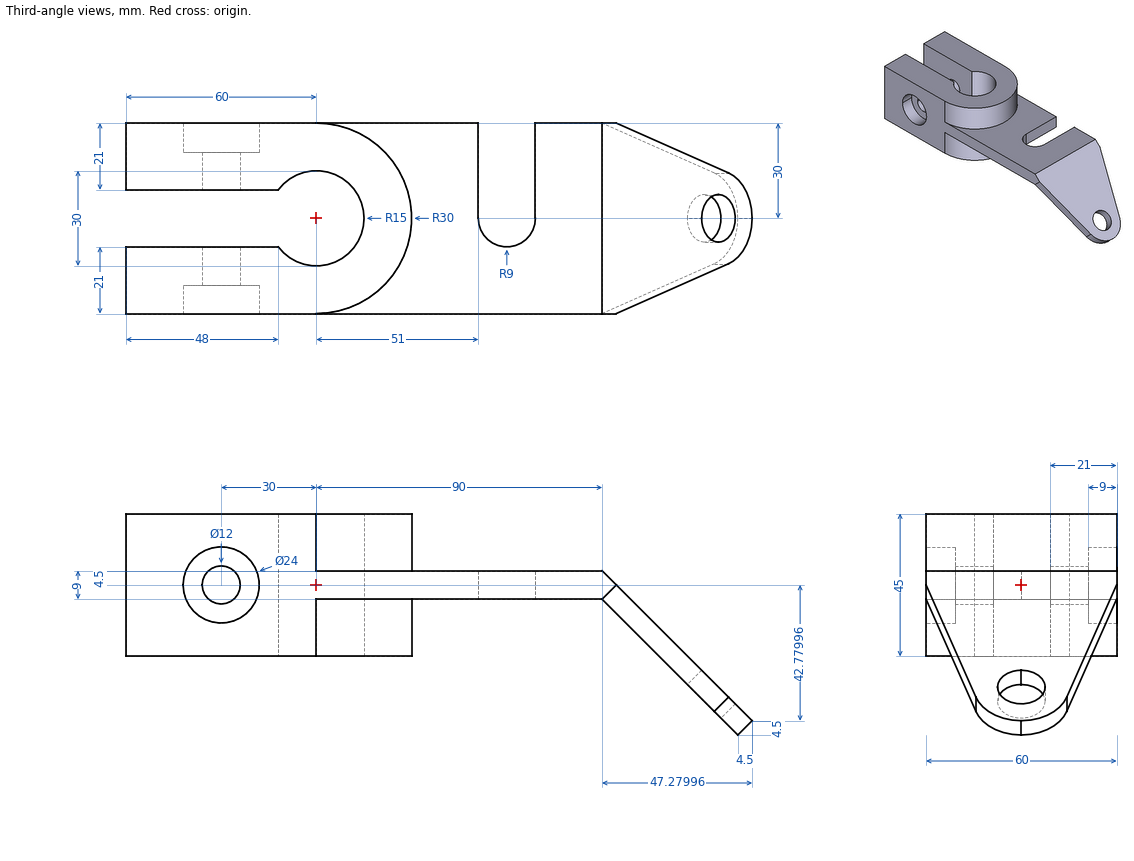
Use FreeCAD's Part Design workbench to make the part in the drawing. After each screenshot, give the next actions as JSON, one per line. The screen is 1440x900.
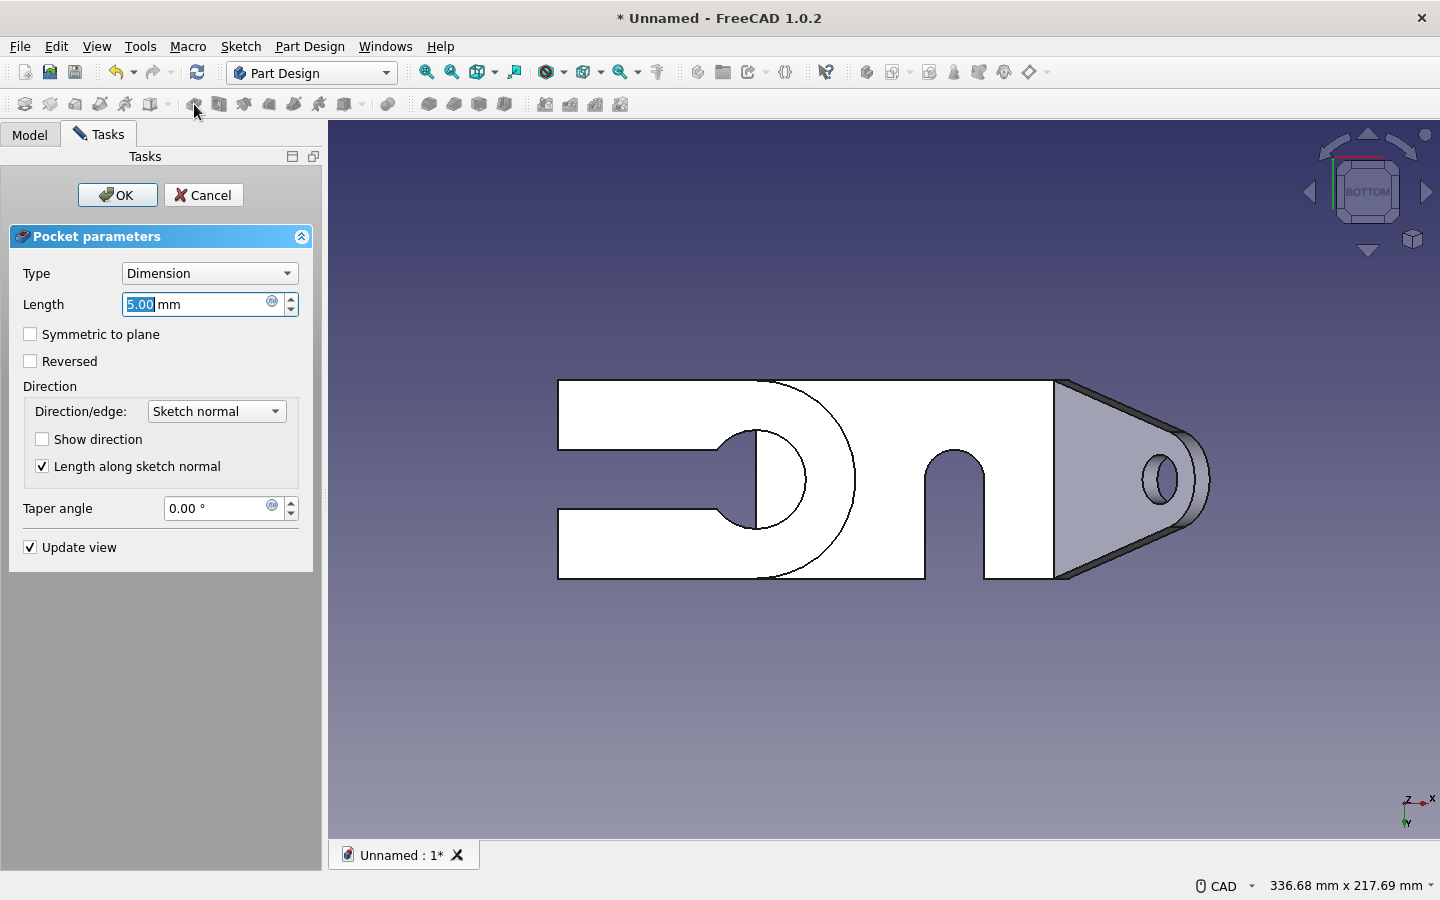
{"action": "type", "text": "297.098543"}
{"action": "key", "text": "Tab"}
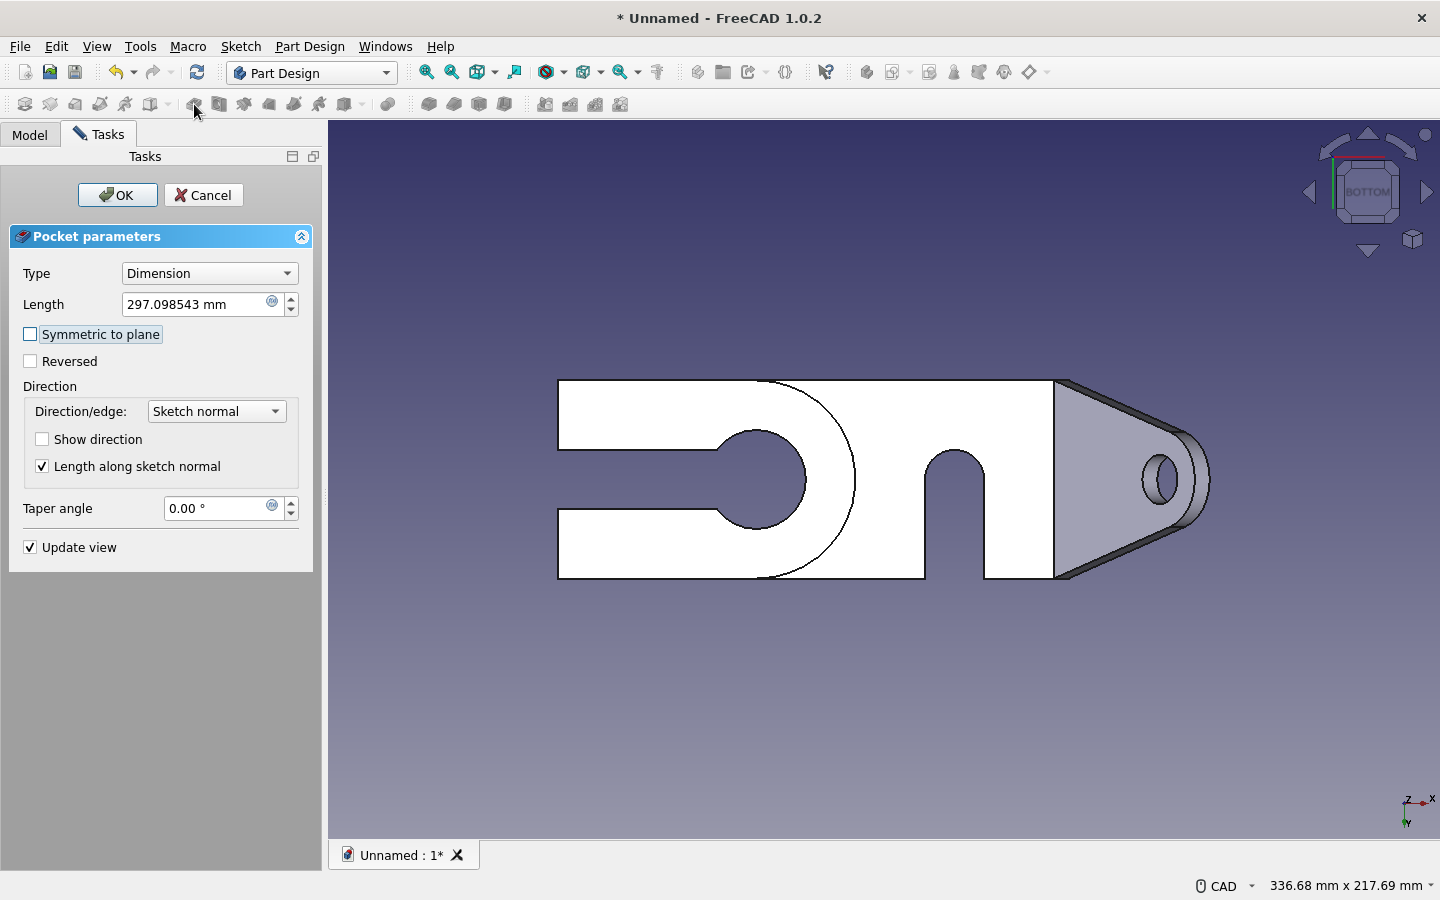
{"action": "left_click", "coordinate": [31, 334]}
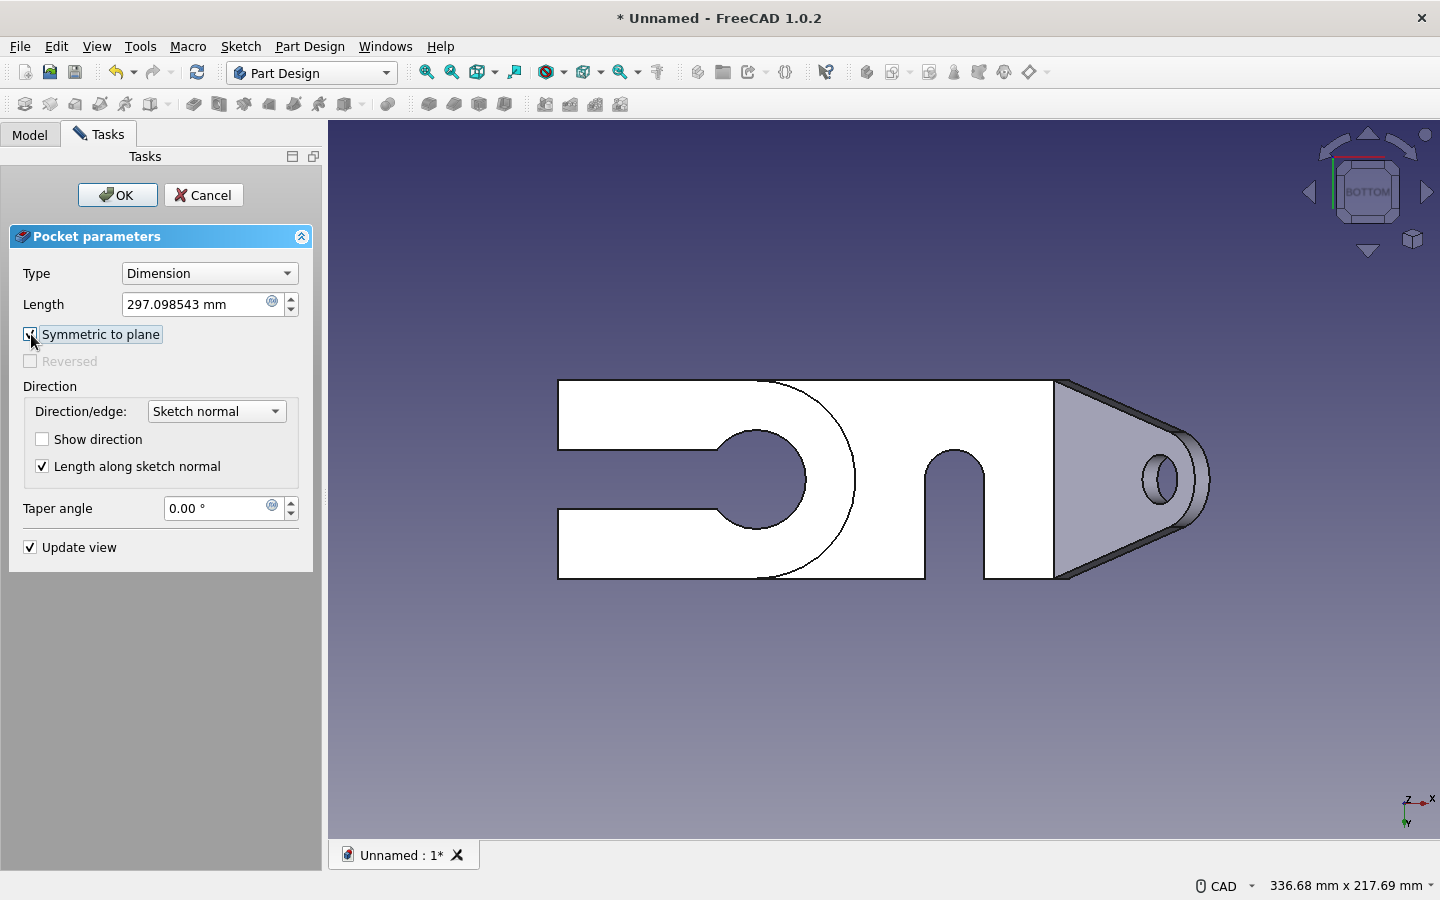
{"action": "left_click", "coordinate": [118, 195]}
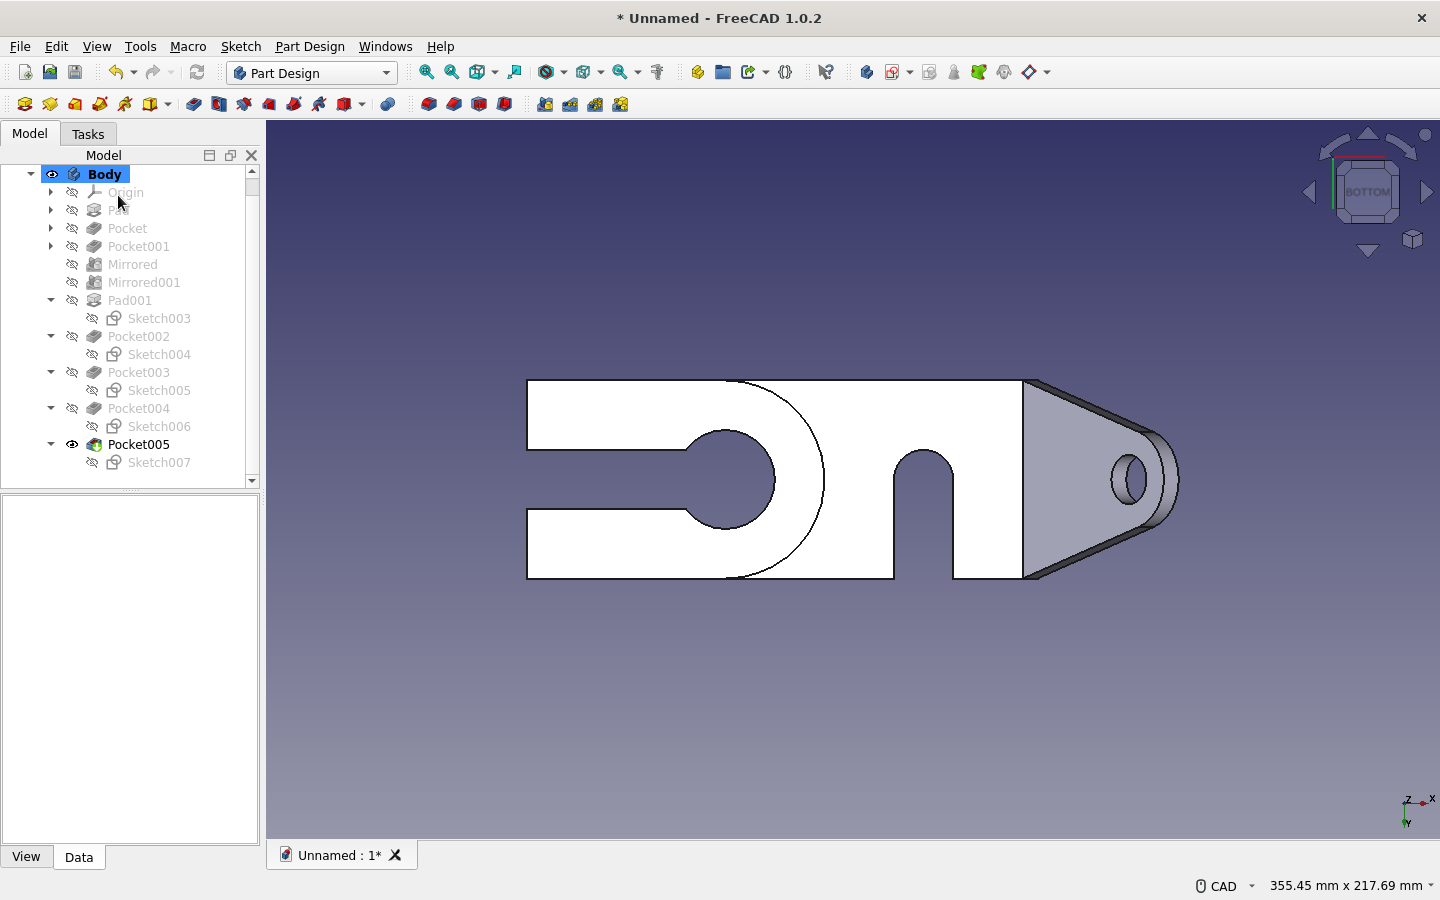
{"action": "key", "text": "0"}